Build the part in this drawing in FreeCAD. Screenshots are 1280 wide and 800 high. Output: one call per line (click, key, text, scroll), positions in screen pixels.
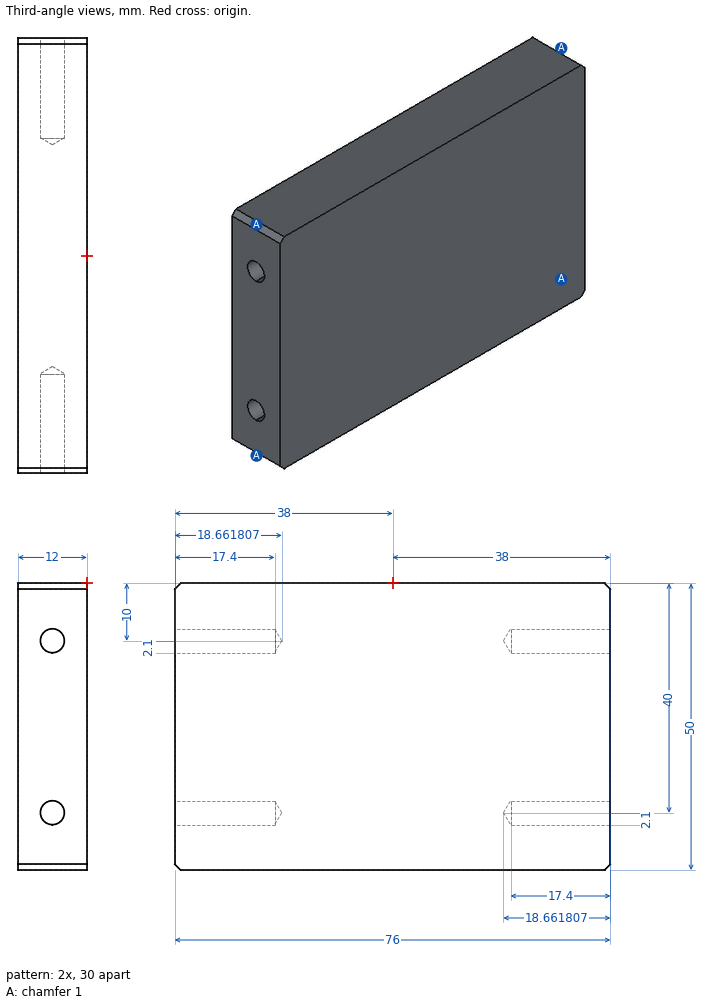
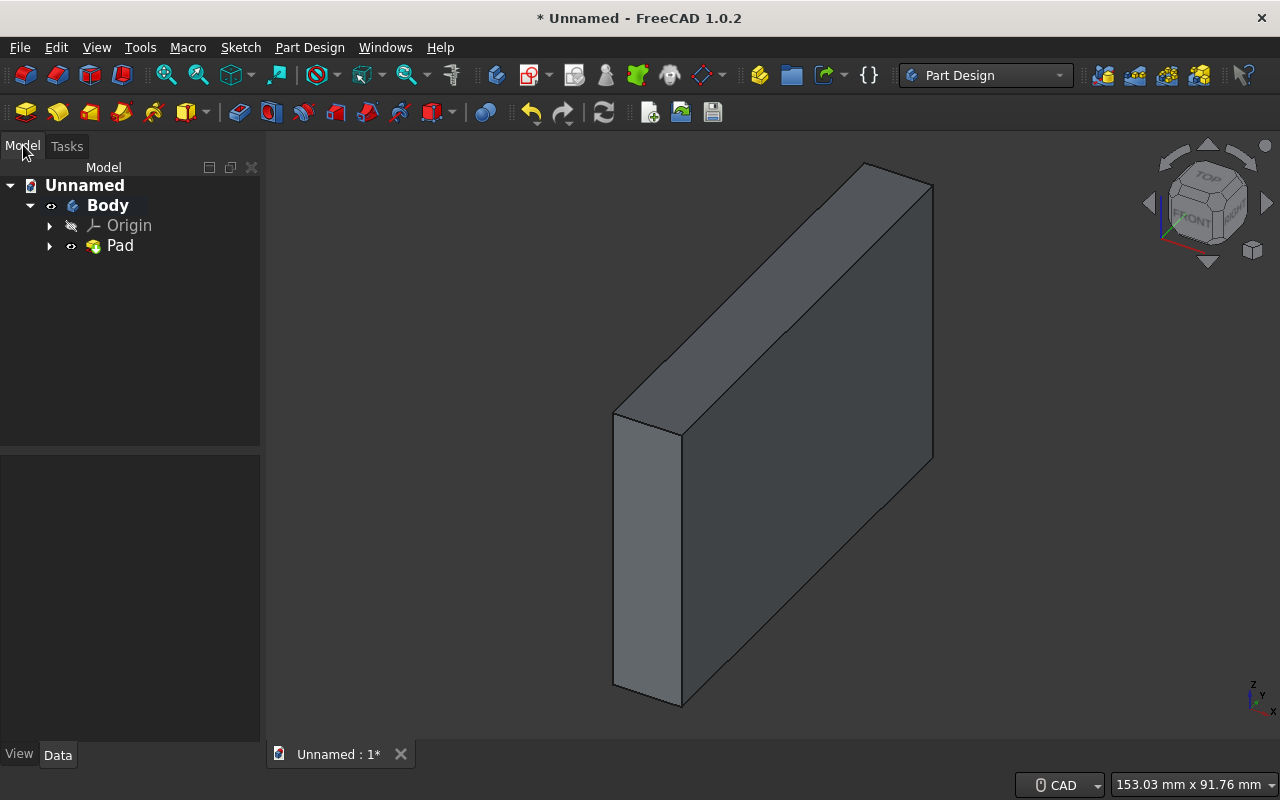
click(50, 226)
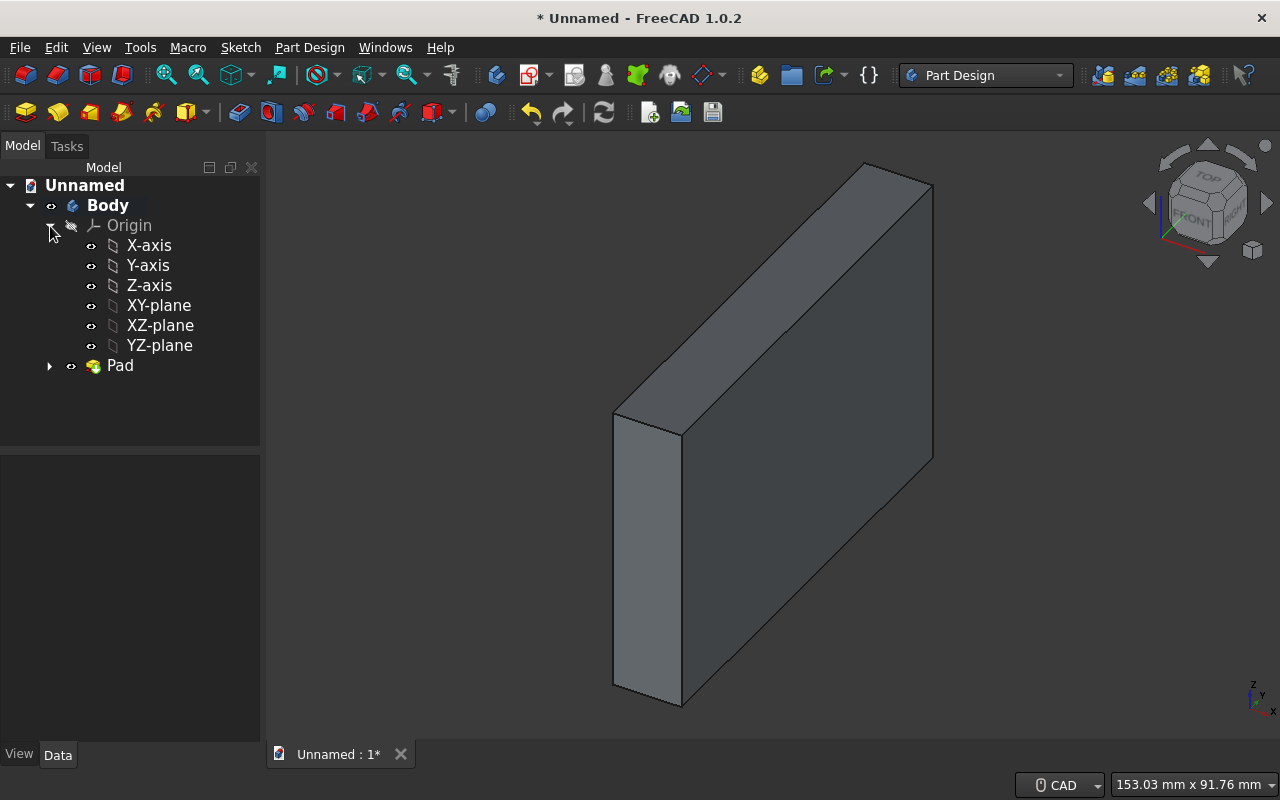
click(136, 346)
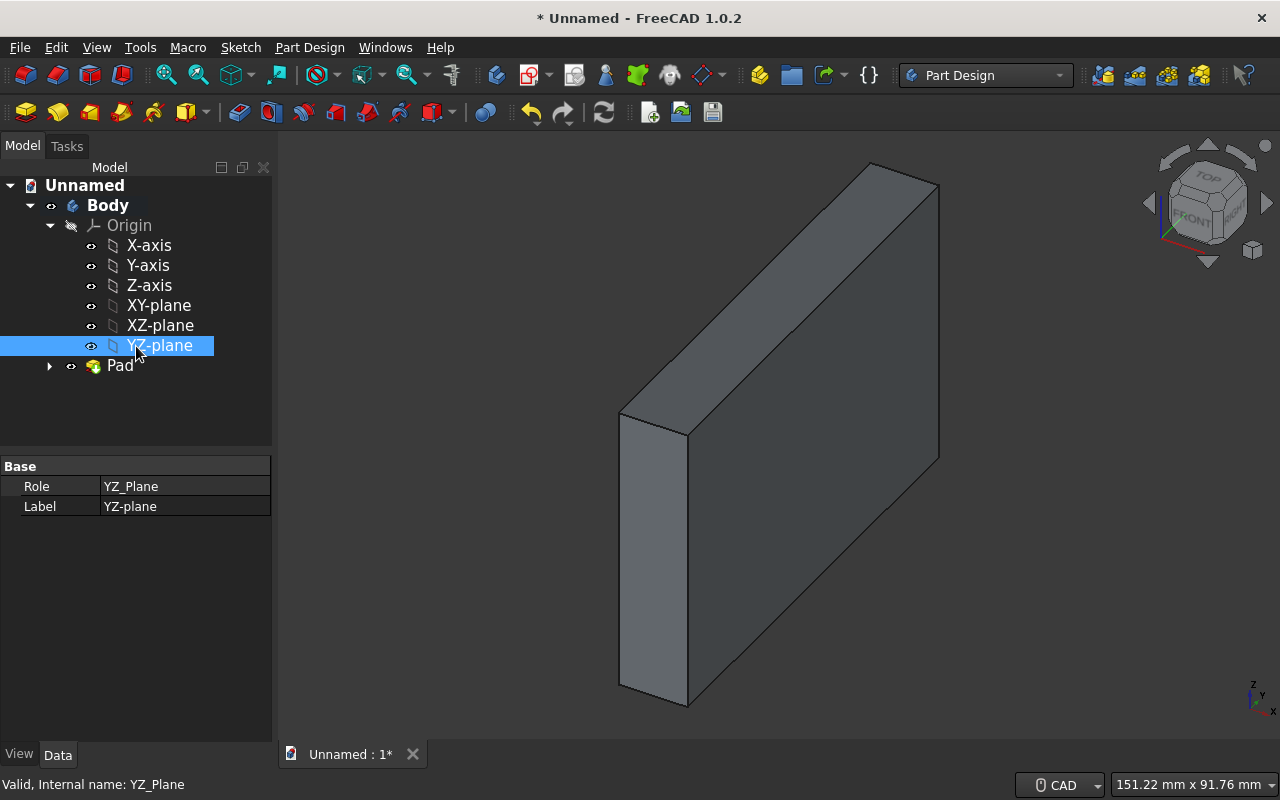
click(702, 76)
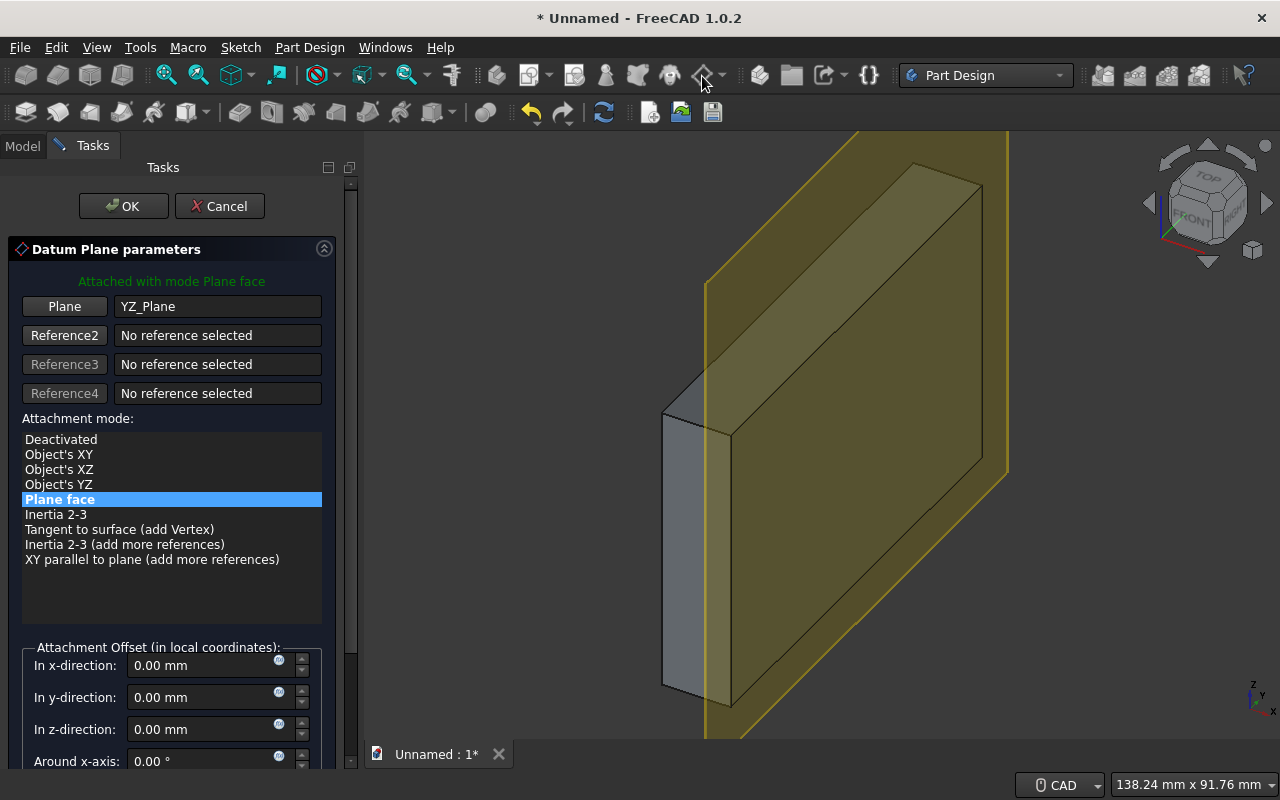
triple_click(210, 729)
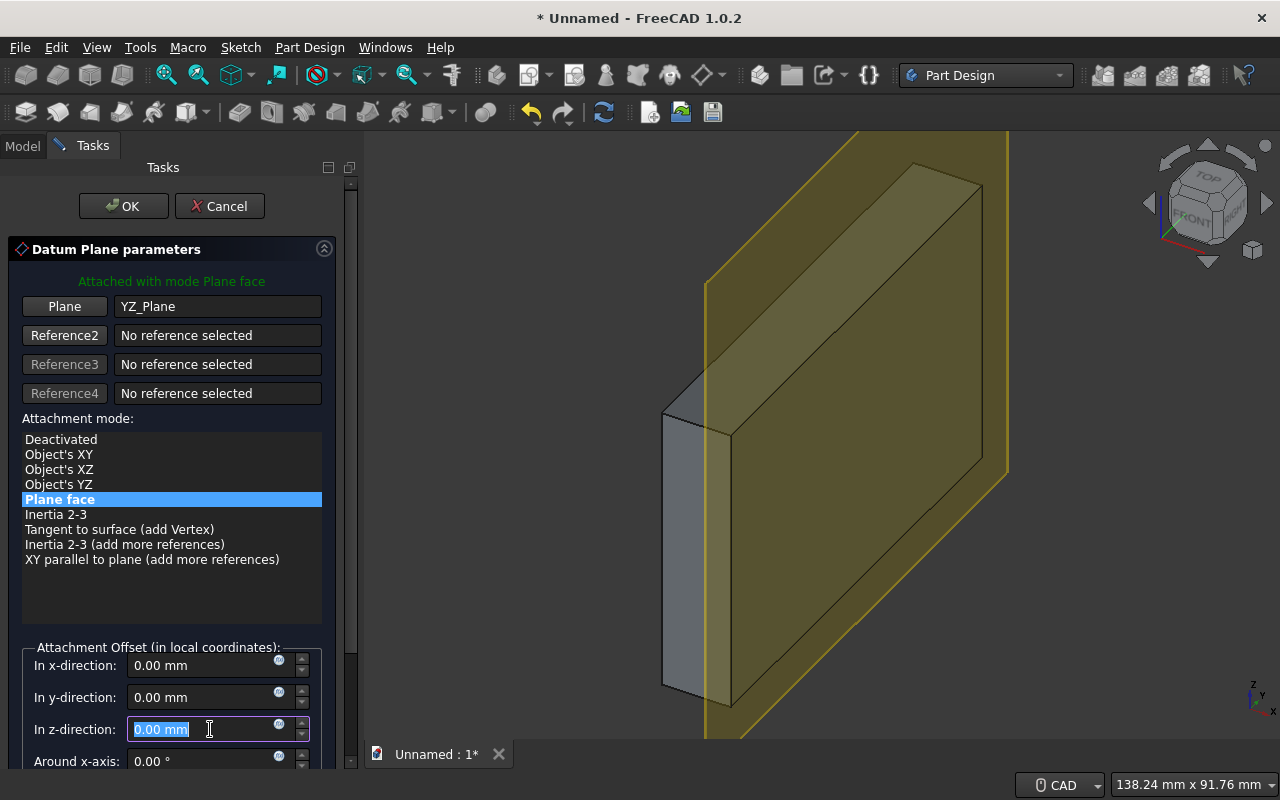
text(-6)
key(Tab)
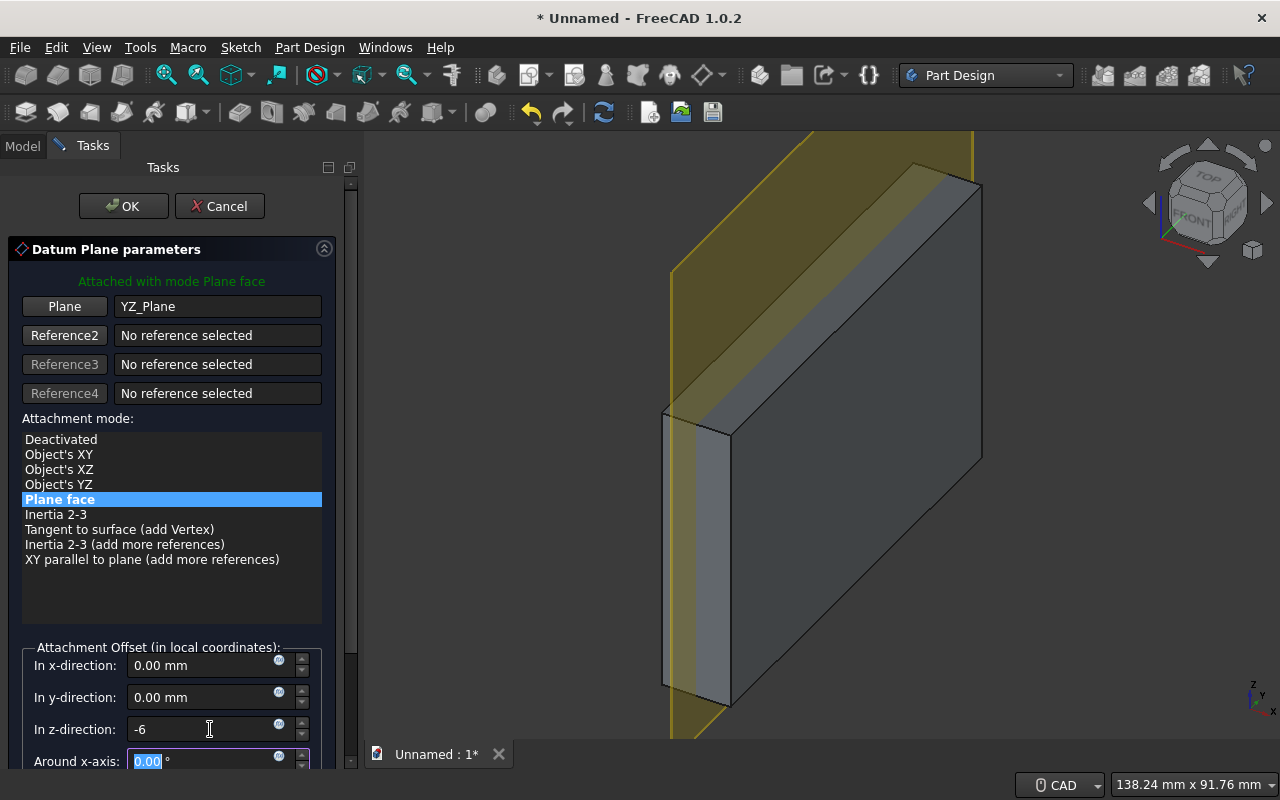
click(124, 206)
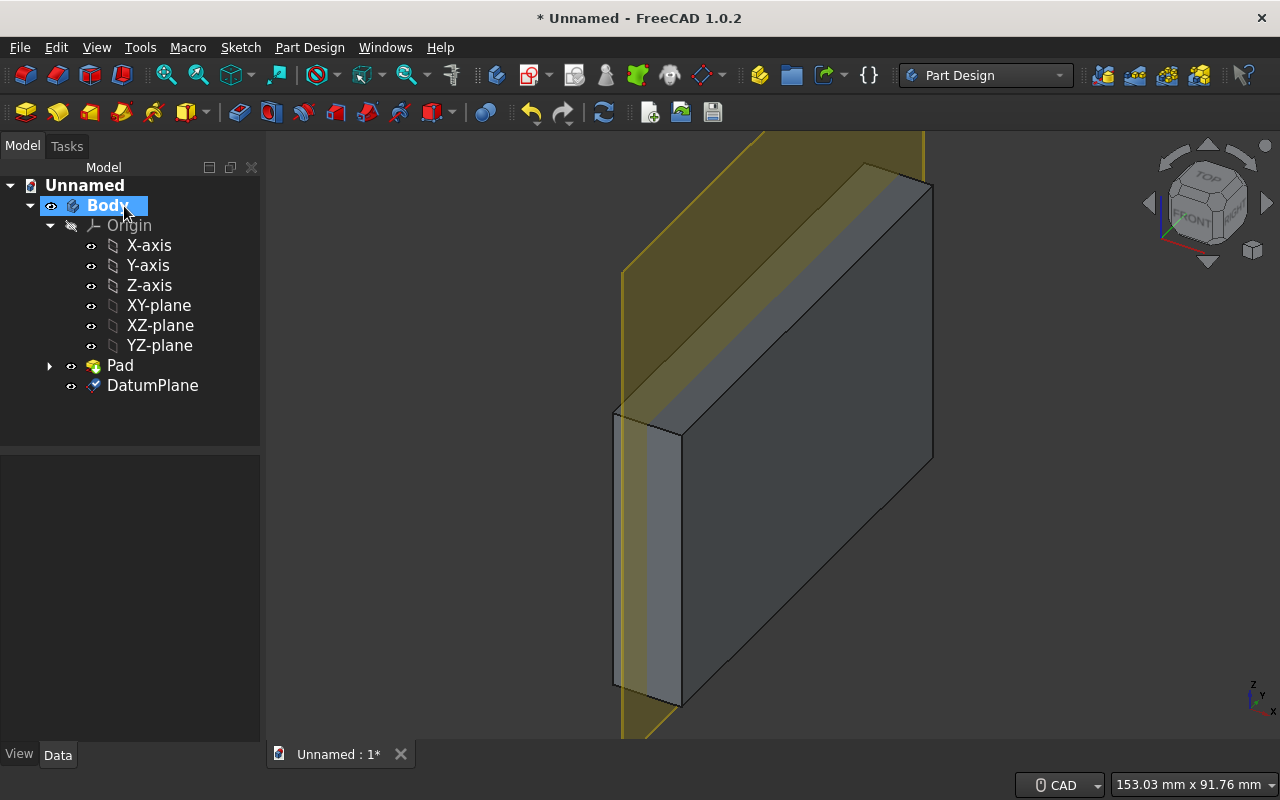
click(116, 386)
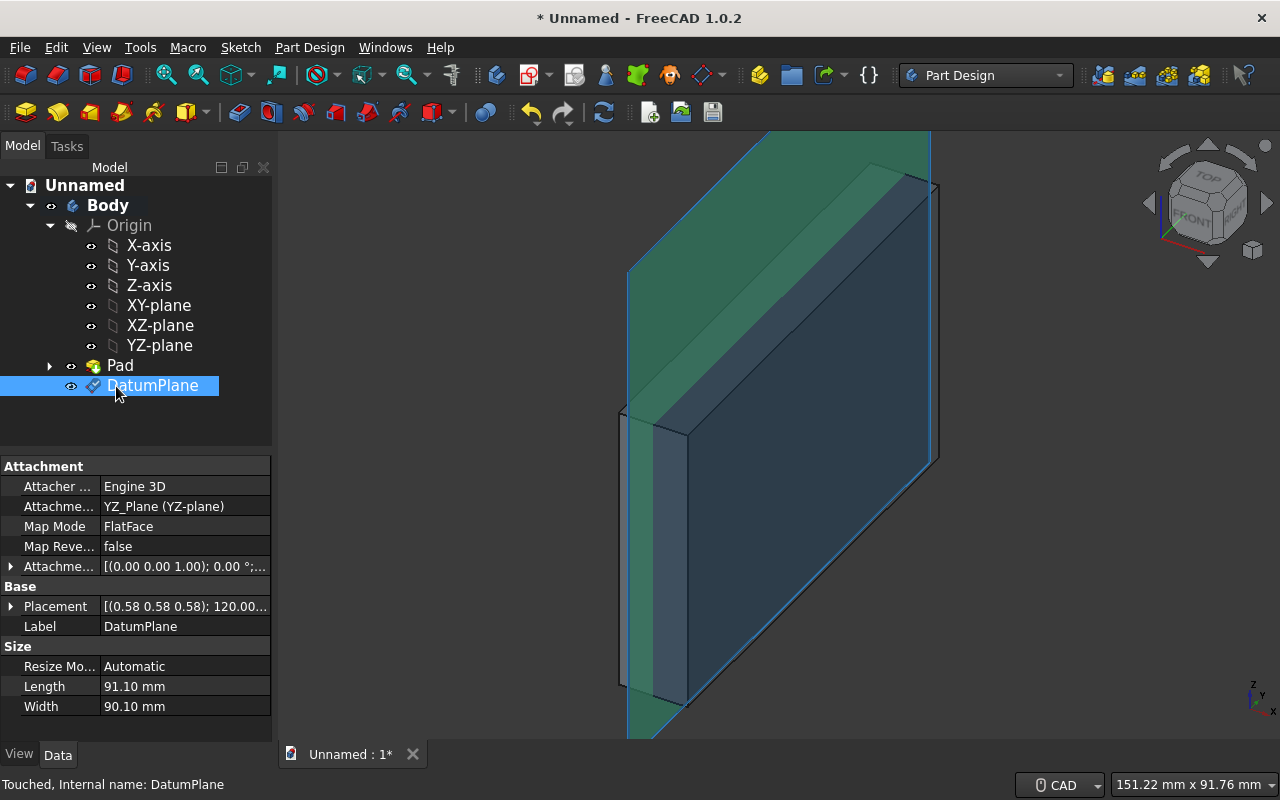
click(530, 76)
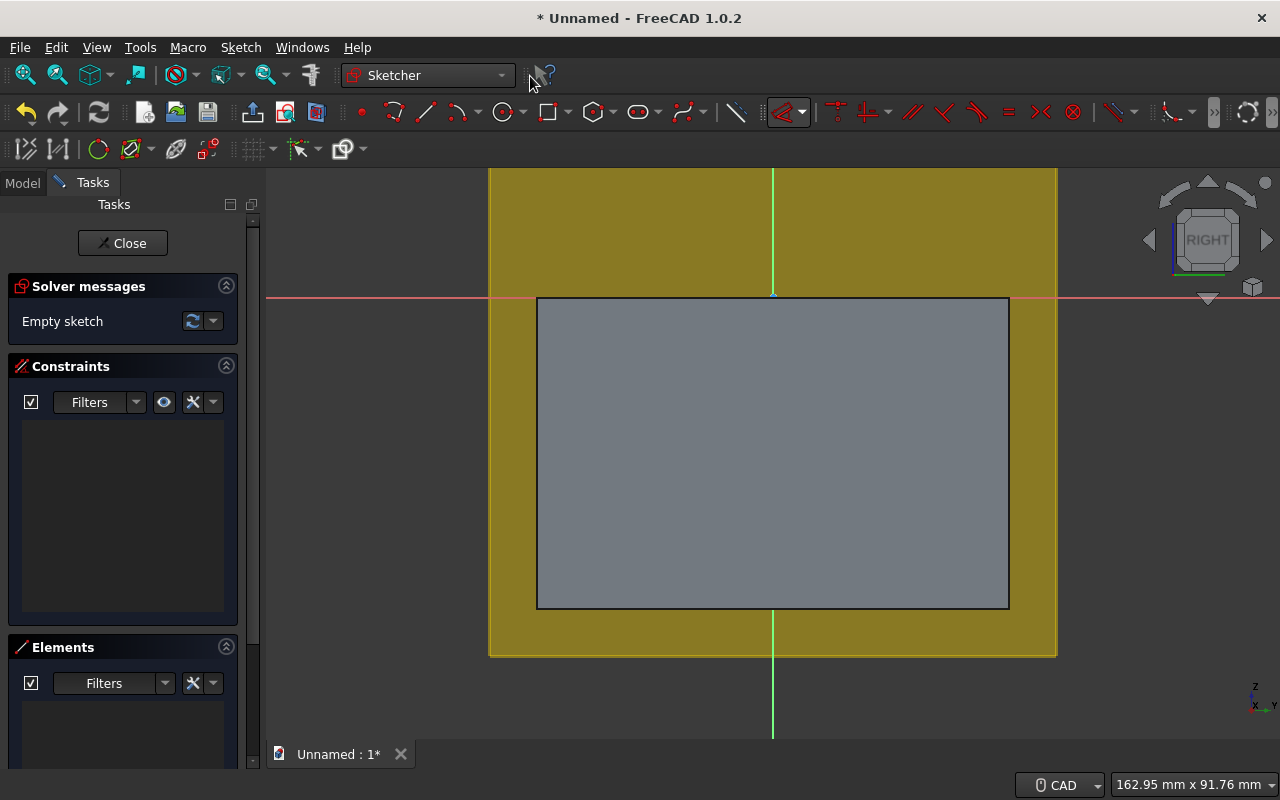
click(318, 112)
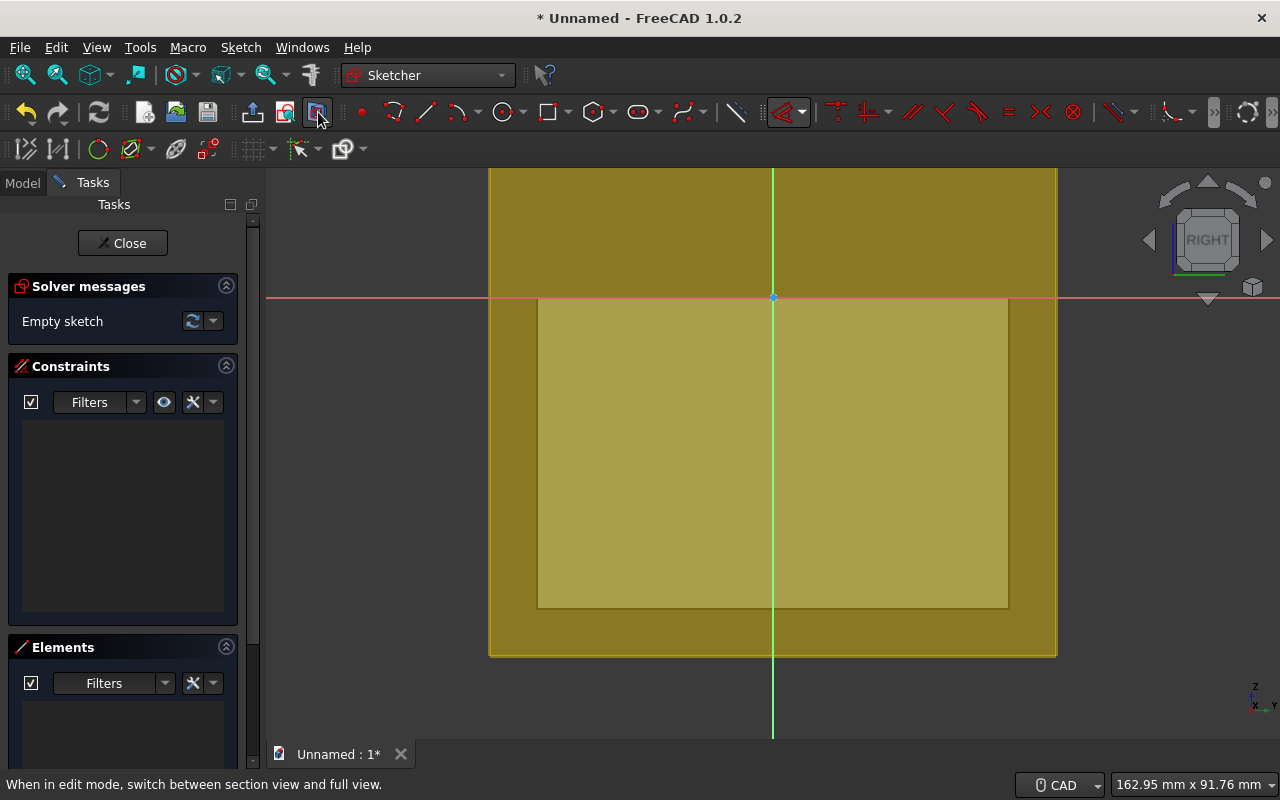
scroll(614, 239, up, 4)